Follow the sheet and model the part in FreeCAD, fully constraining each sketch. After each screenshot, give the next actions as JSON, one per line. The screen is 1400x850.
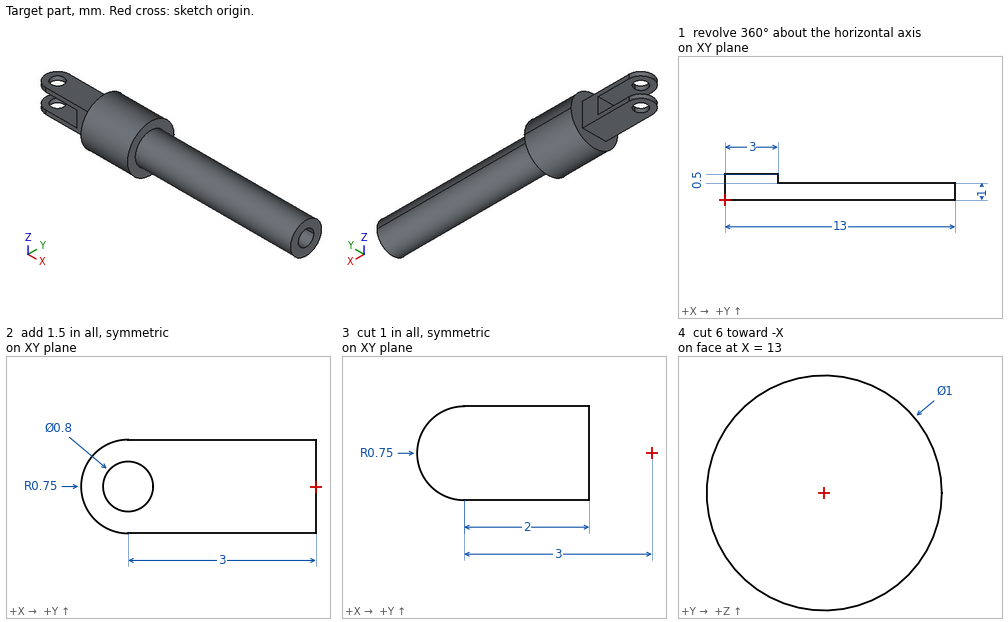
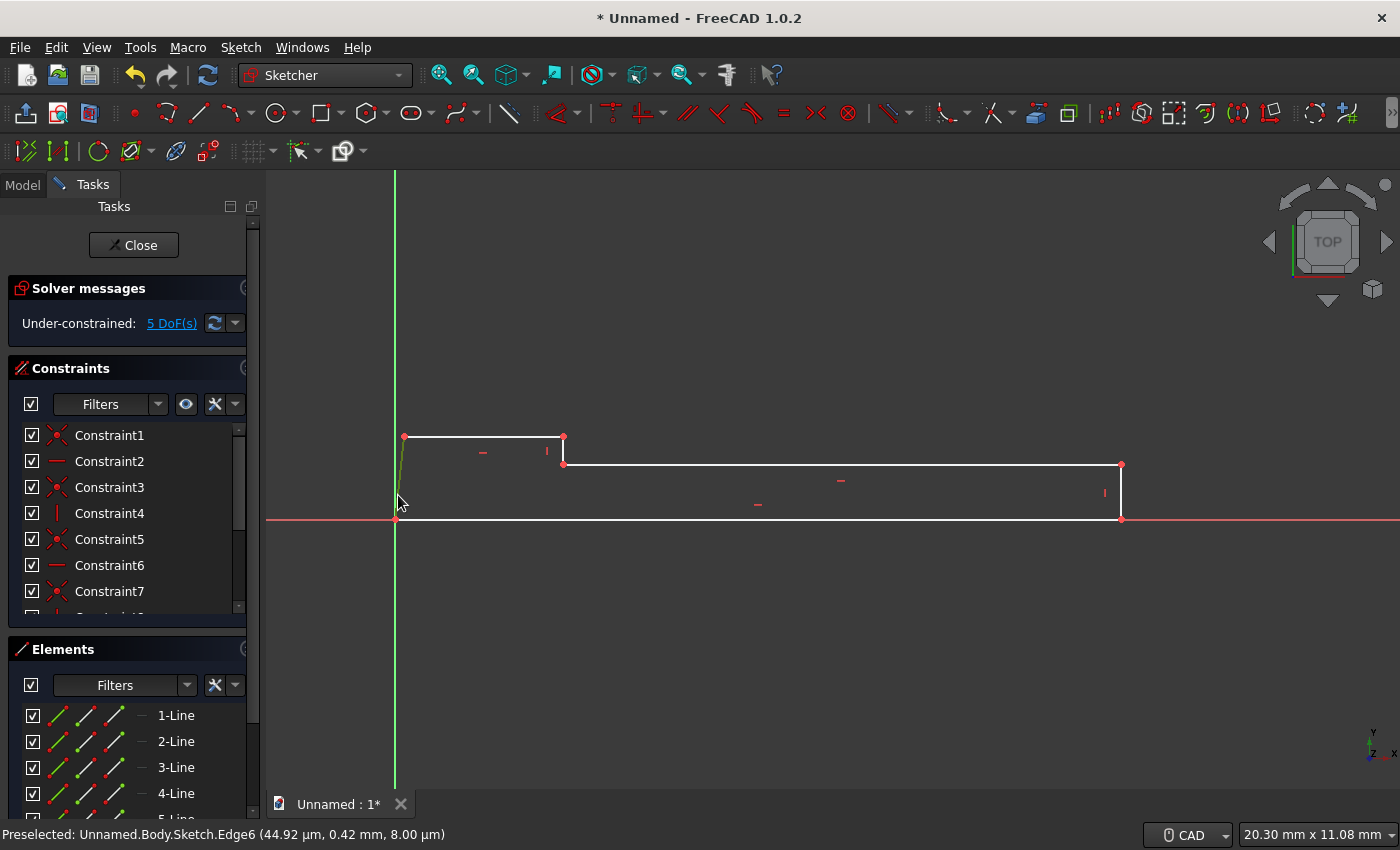
{"action": "left_click", "coordinate": [666, 114]}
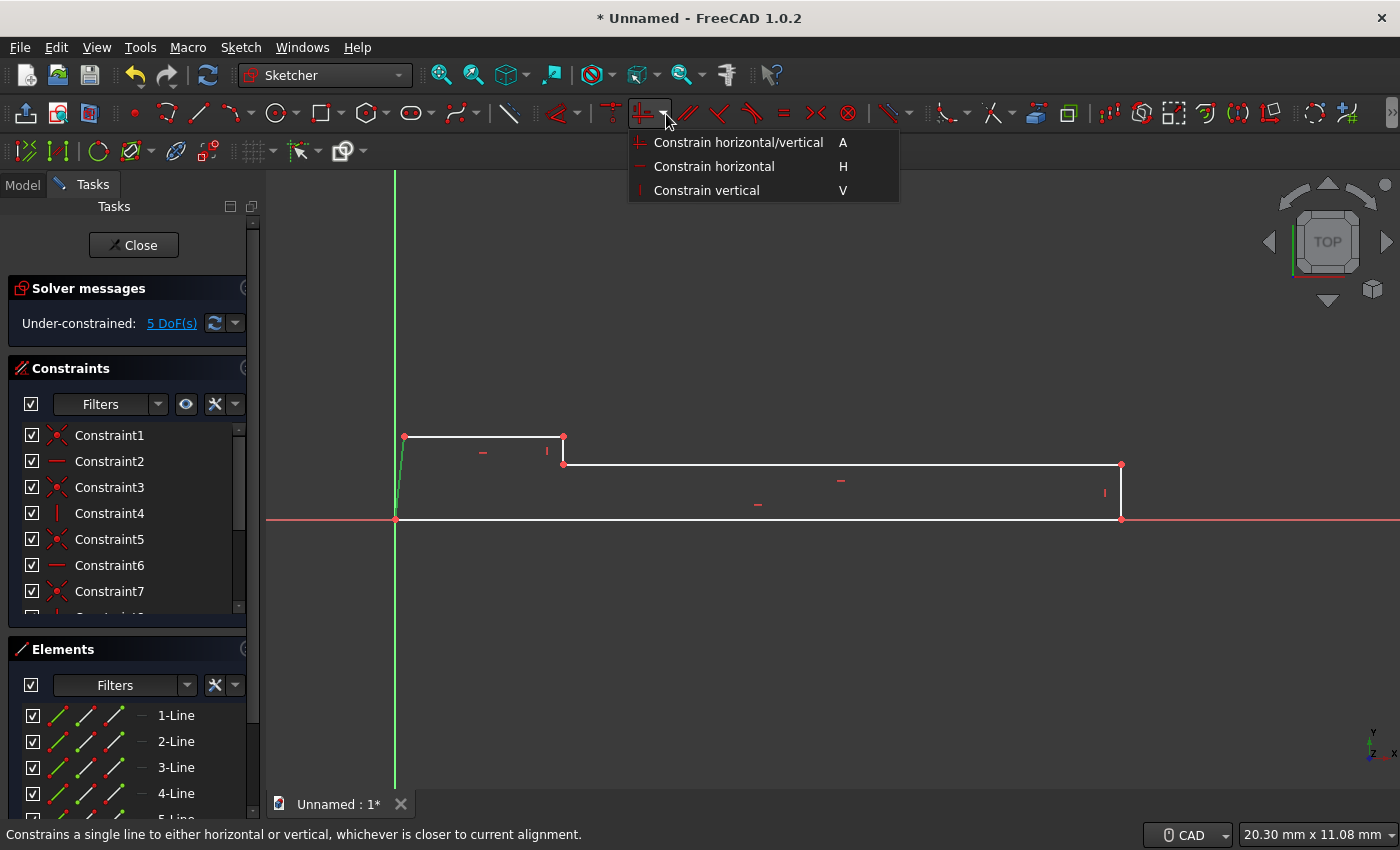
{"action": "left_click", "coordinate": [764, 190]}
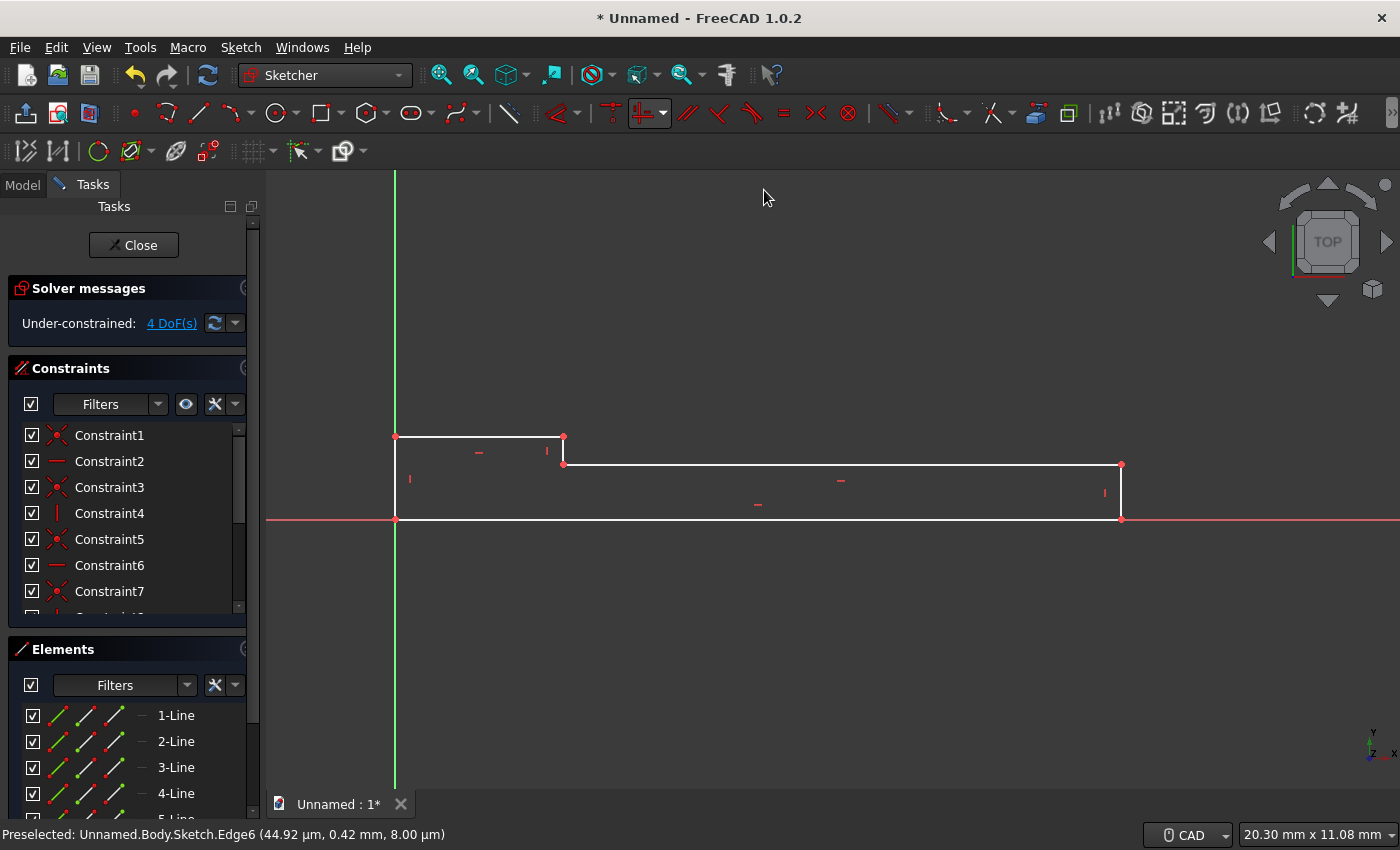
{"action": "key", "text": "d"}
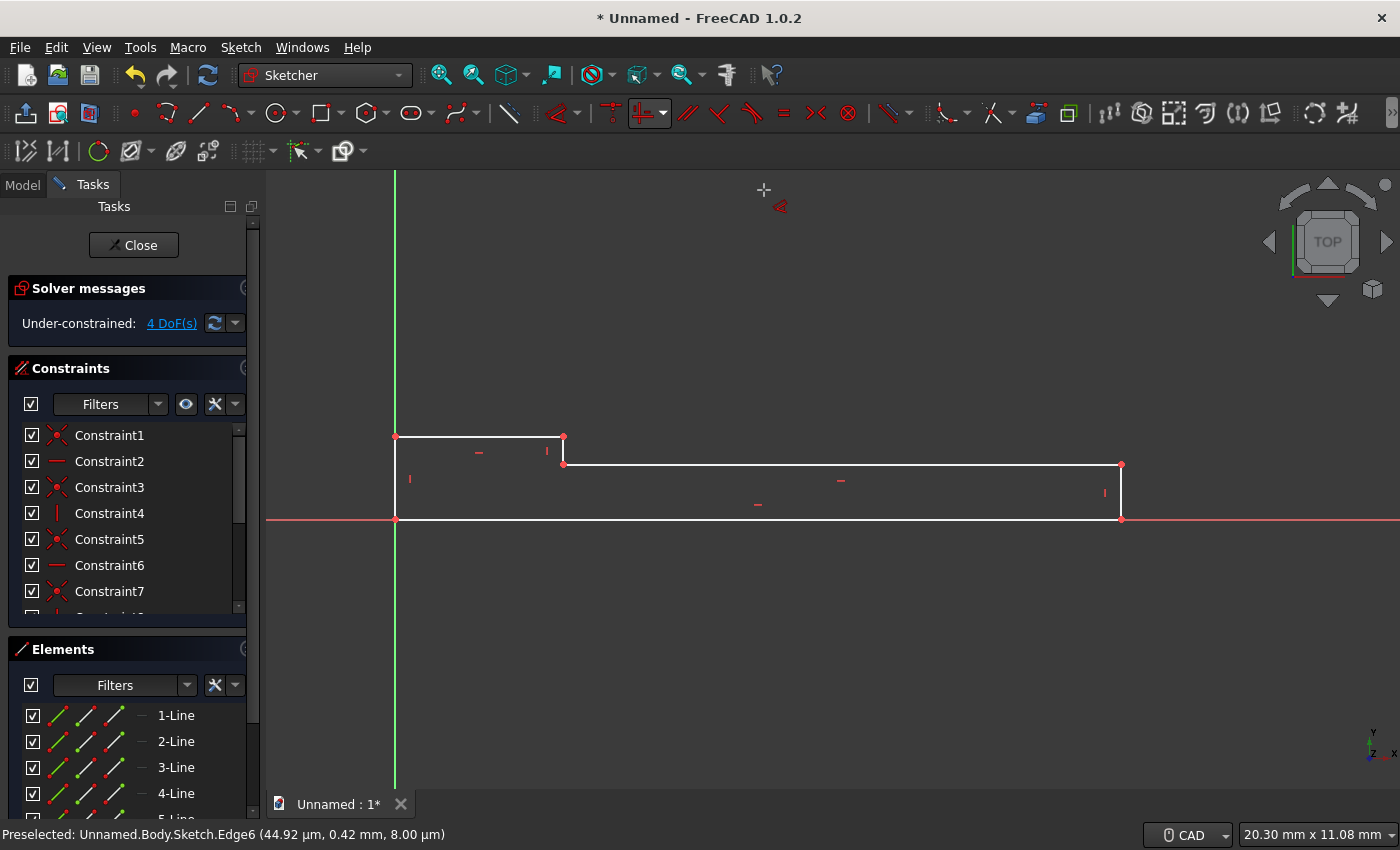
{"action": "left_click", "coordinate": [1121, 503]}
{"action": "left_click", "coordinate": [1155, 492]}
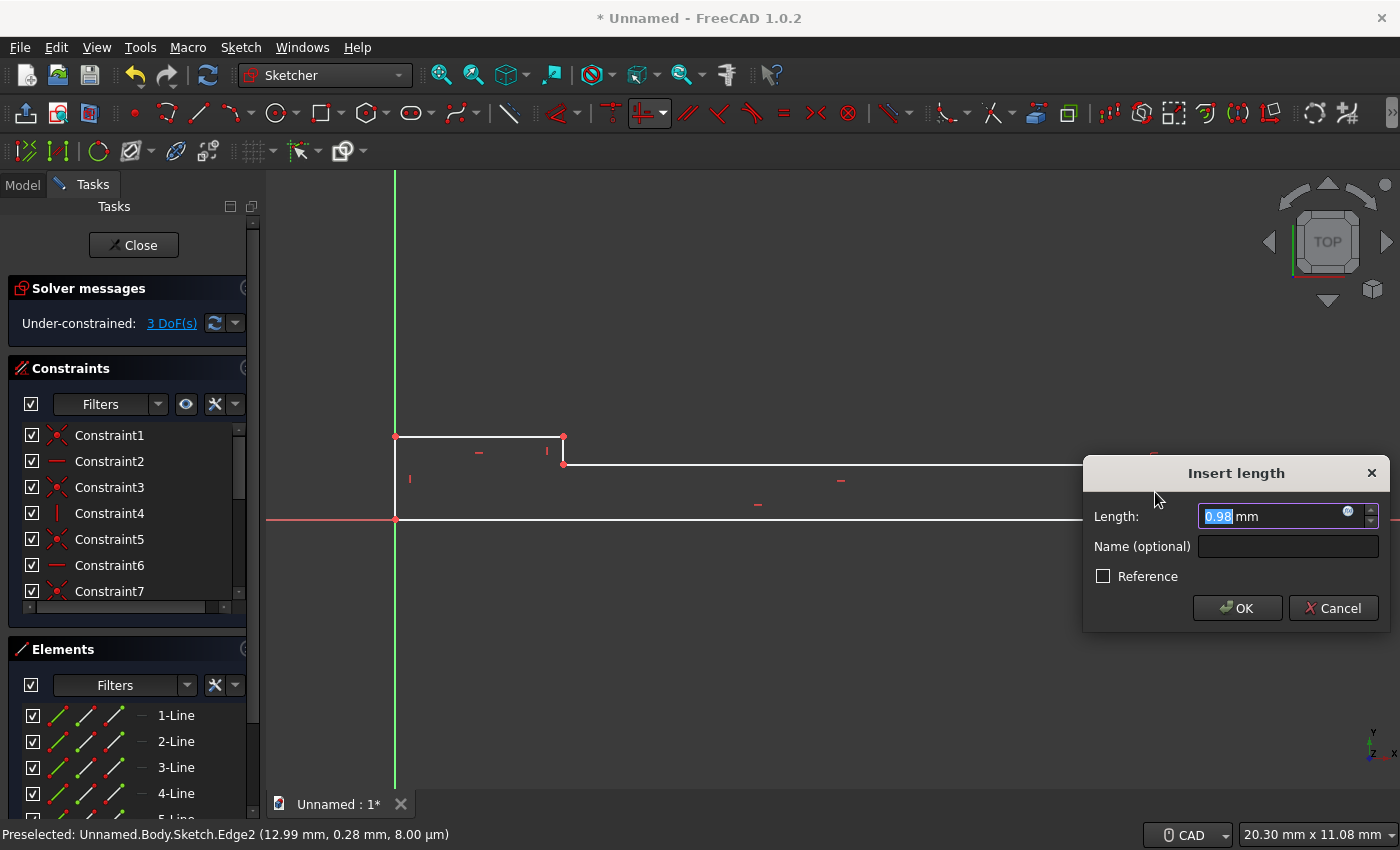
{"action": "type", "text": "1"}
{"action": "key", "text": "Return"}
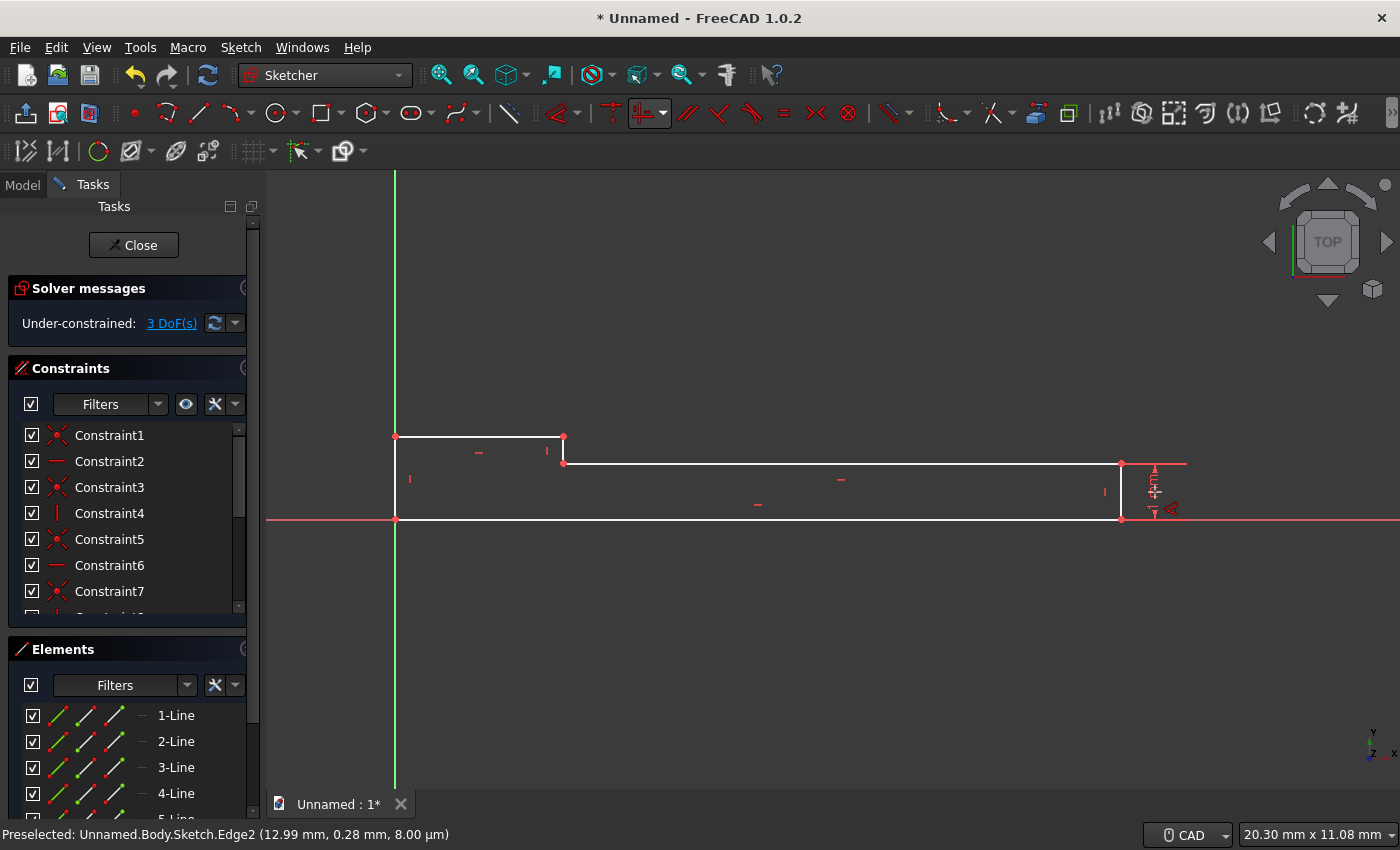
{"action": "left_click", "coordinate": [513, 437]}
{"action": "left_click", "coordinate": [479, 403]}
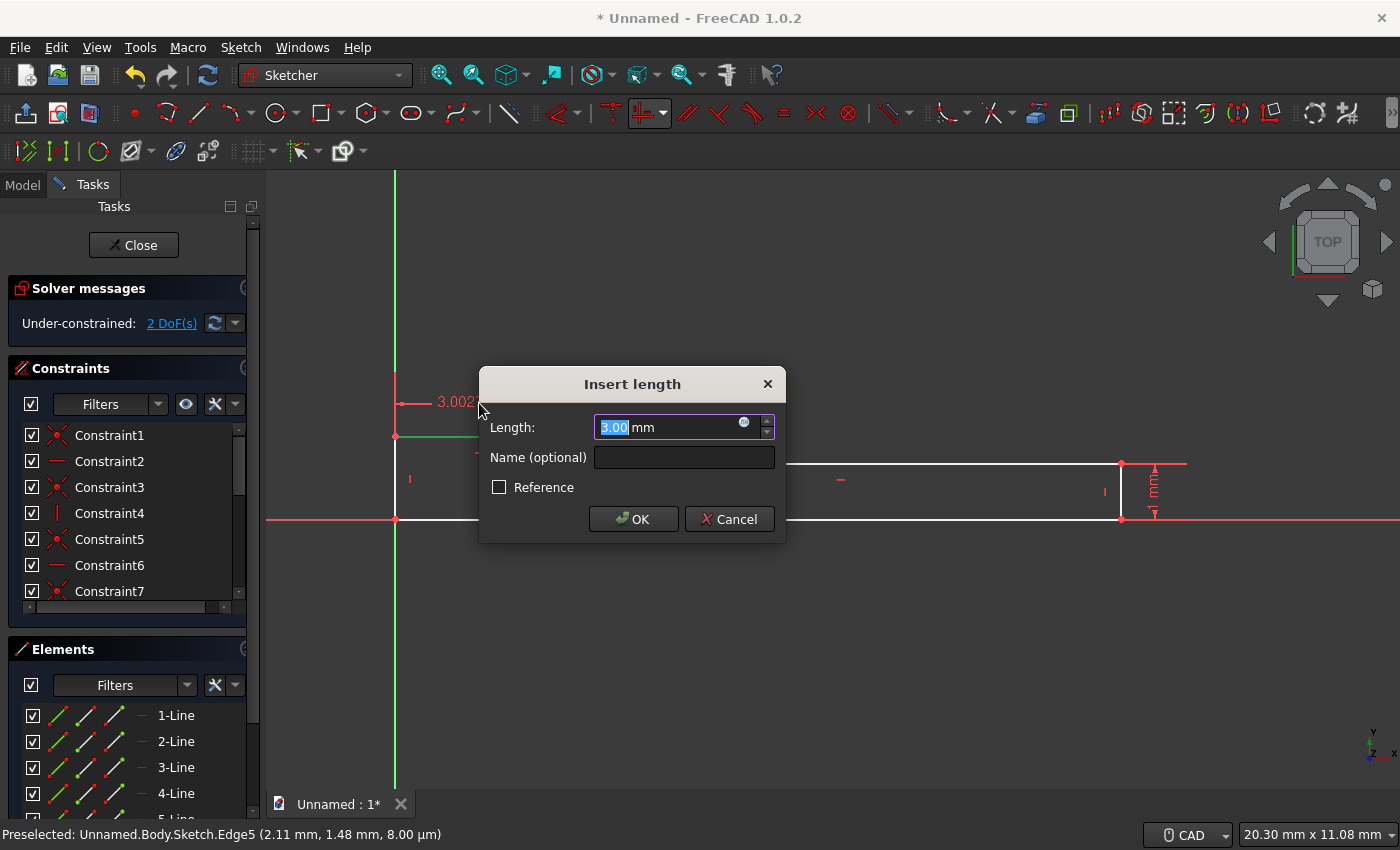
{"action": "type", "text": "3"}
{"action": "key", "text": "Return"}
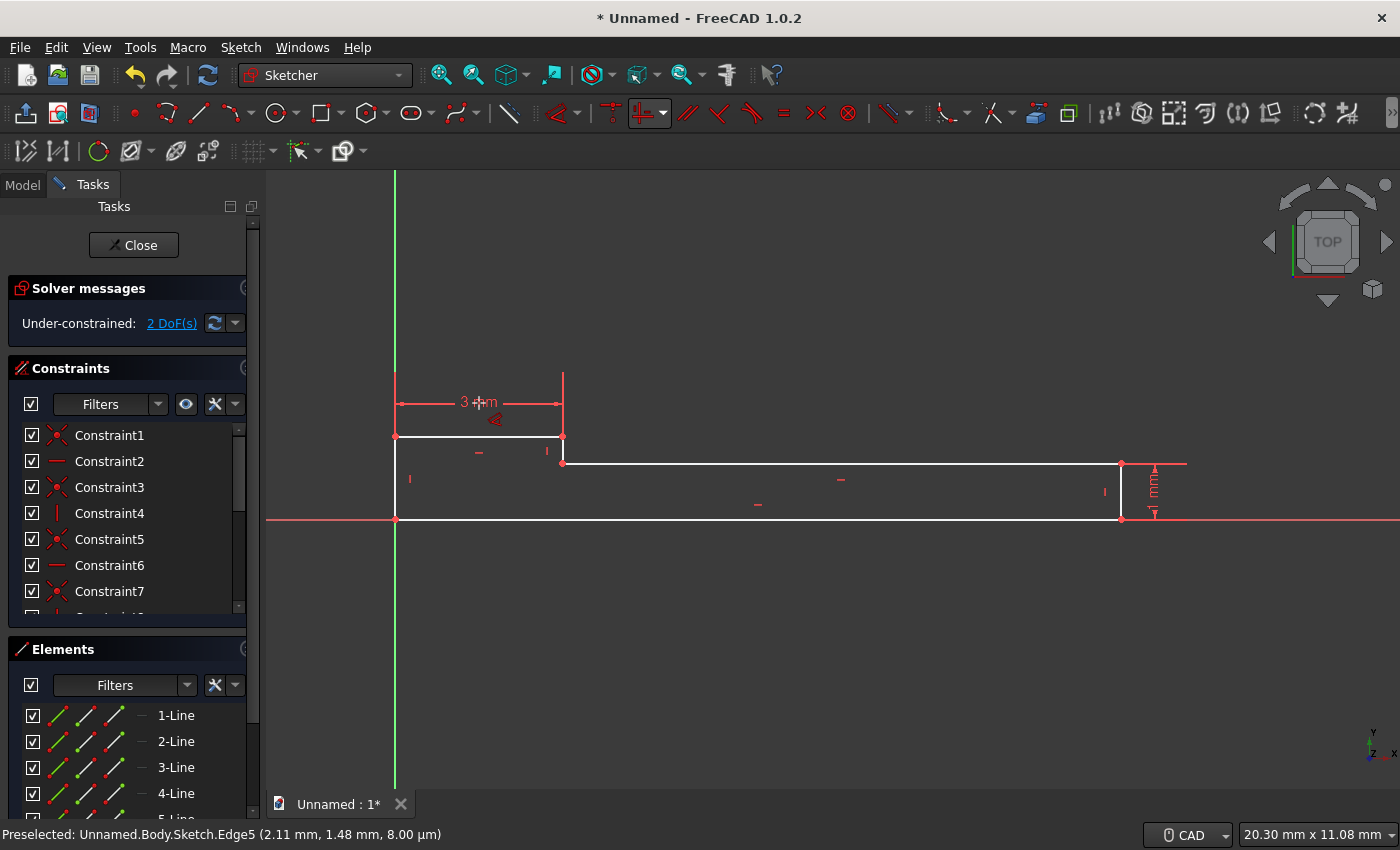
{"action": "left_click", "coordinate": [613, 520]}
{"action": "left_click", "coordinate": [758, 554]}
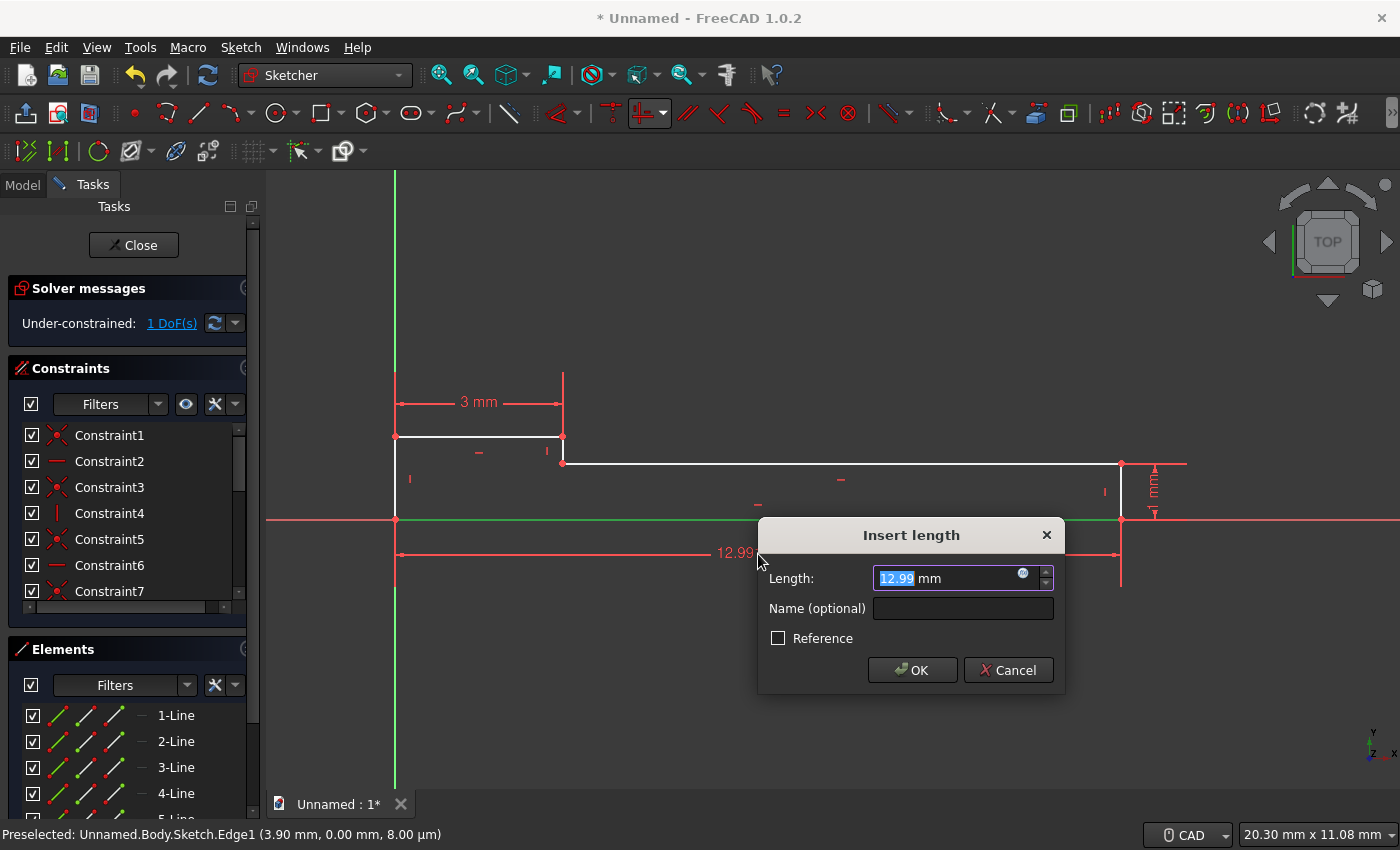
{"action": "type", "text": "13"}
{"action": "key", "text": "Return"}